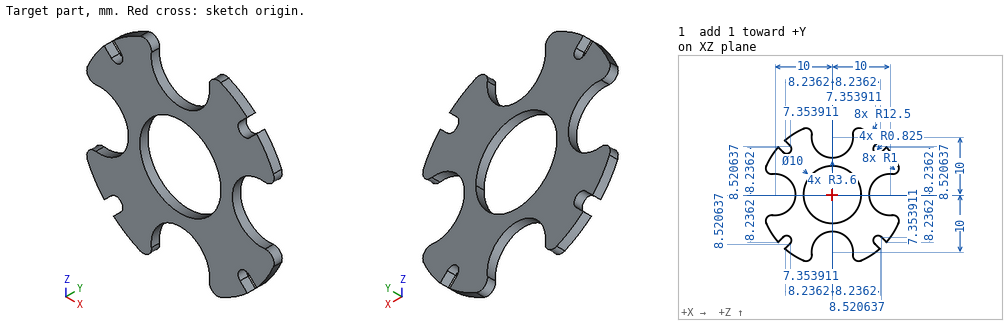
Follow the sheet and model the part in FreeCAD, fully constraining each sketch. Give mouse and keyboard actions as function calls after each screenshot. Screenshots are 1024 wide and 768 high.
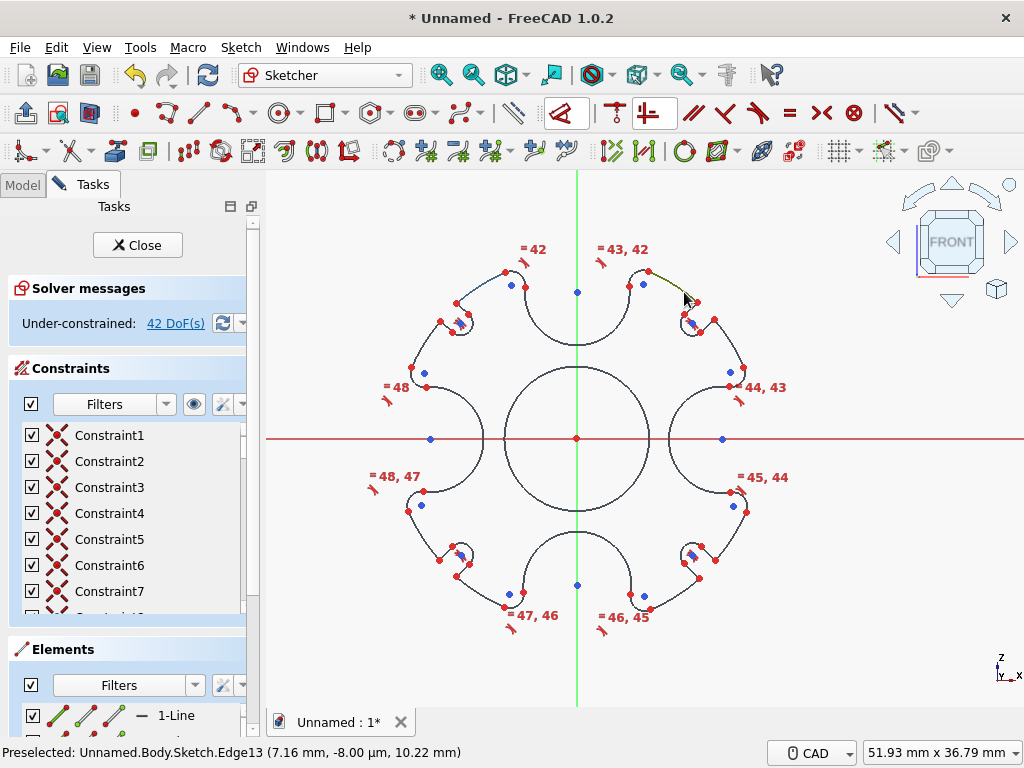
click(737, 352)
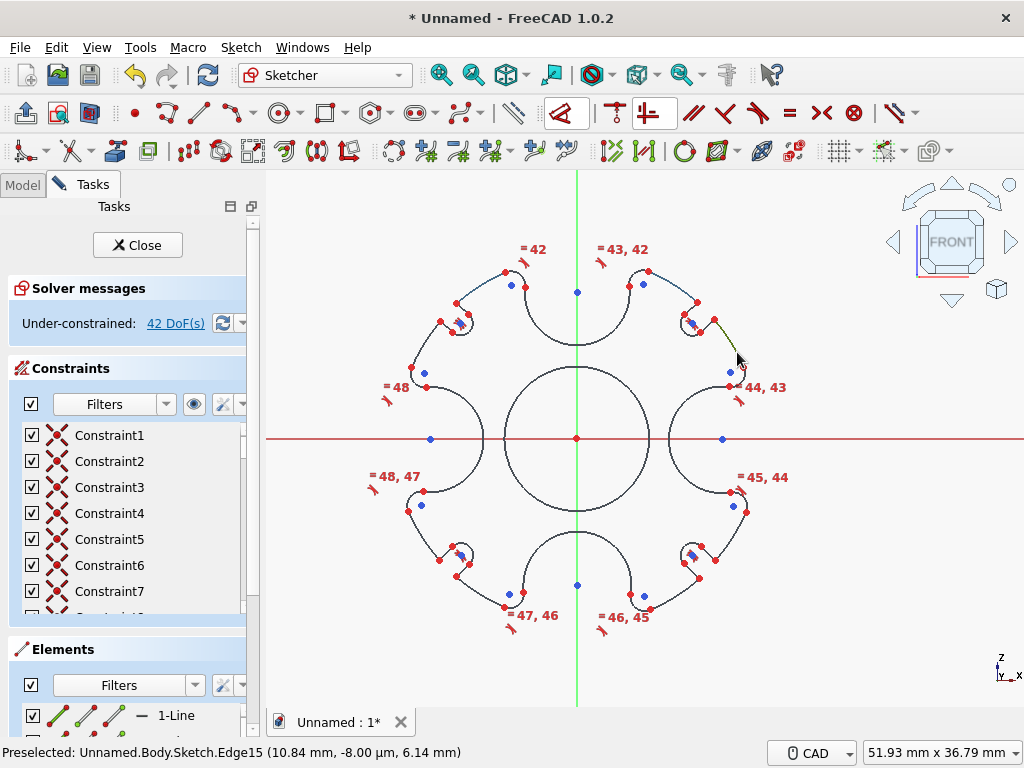
click(726, 547)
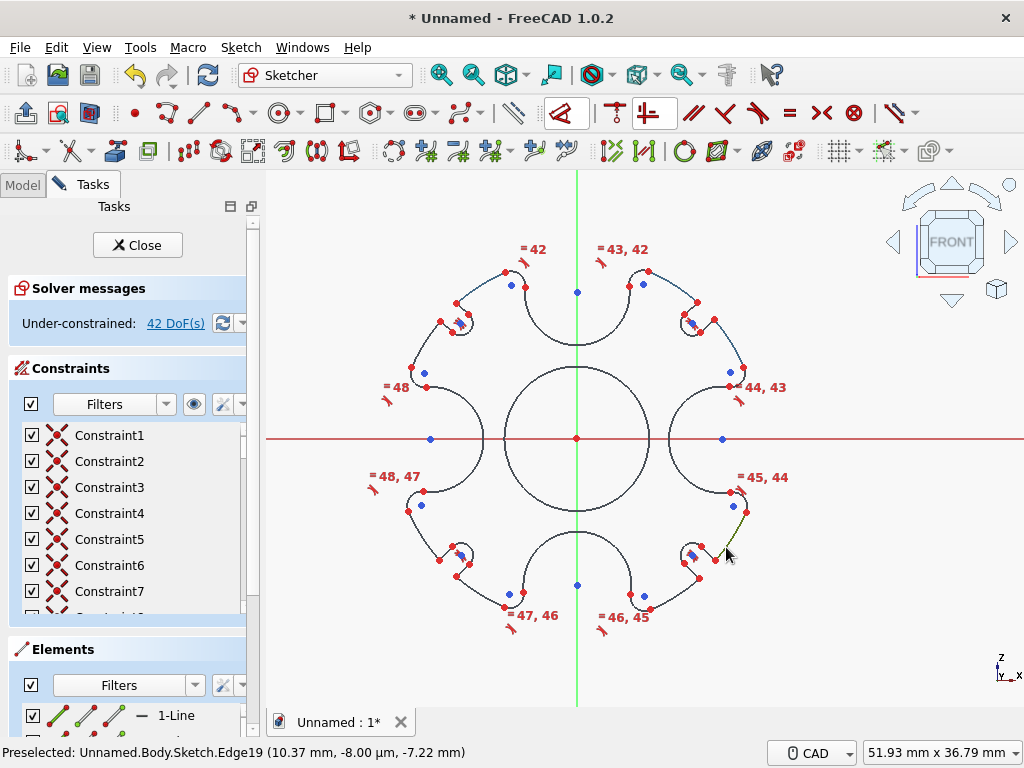
click(666, 602)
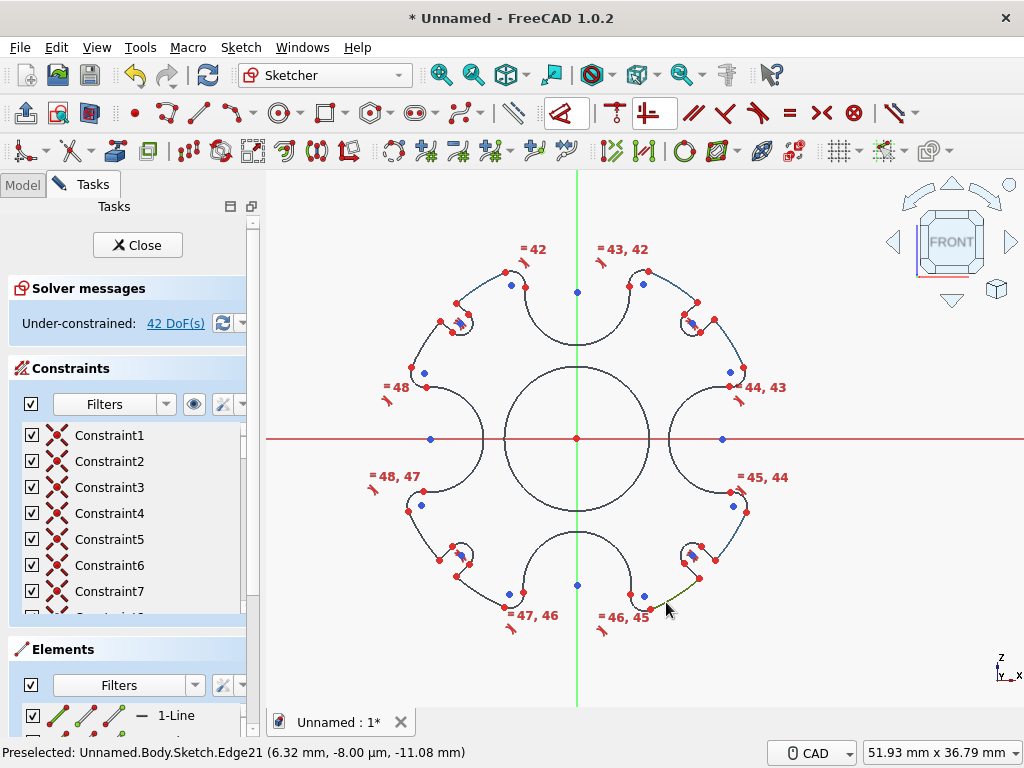
click(470, 588)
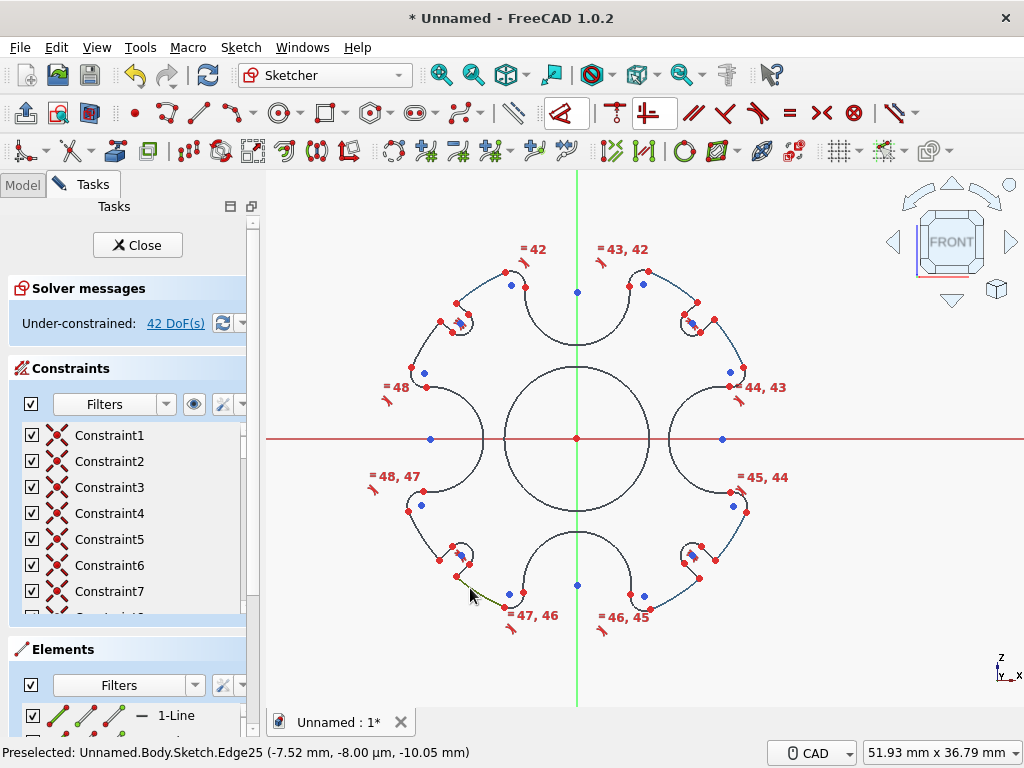
click(416, 527)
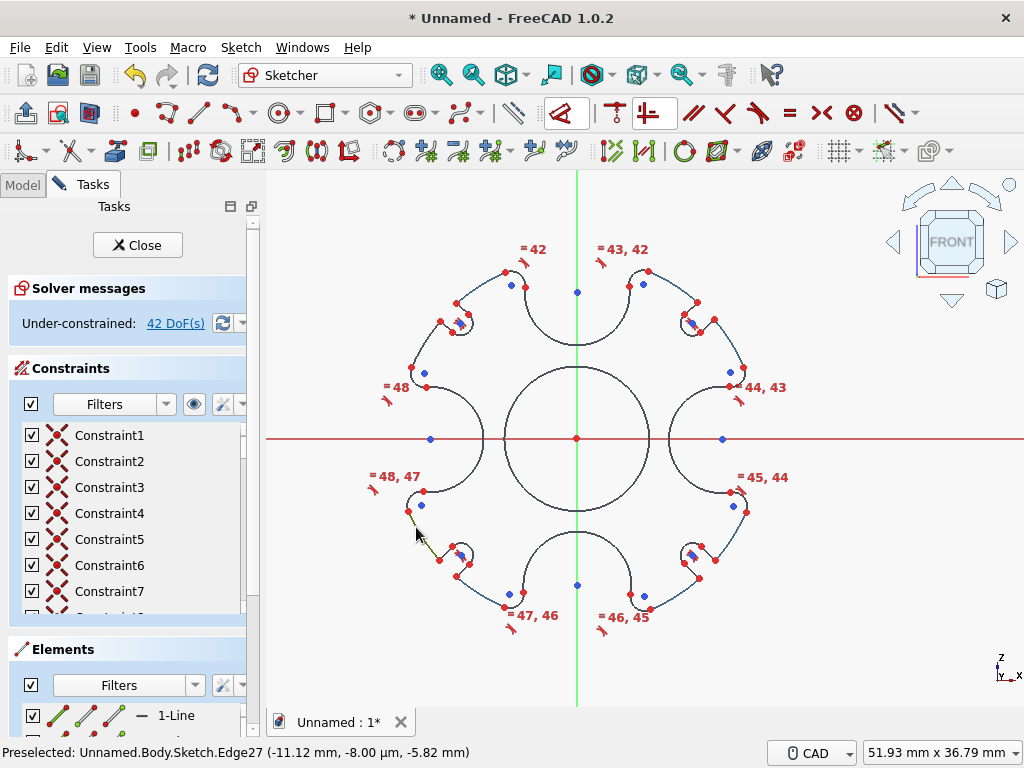
click(431, 334)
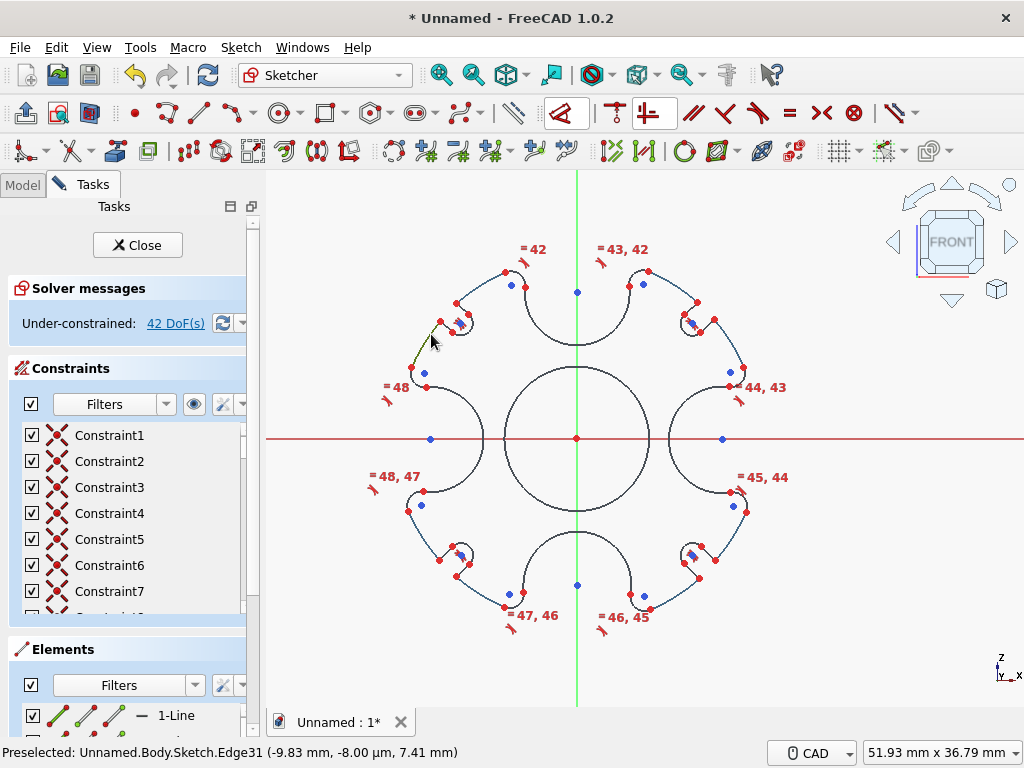
key(e)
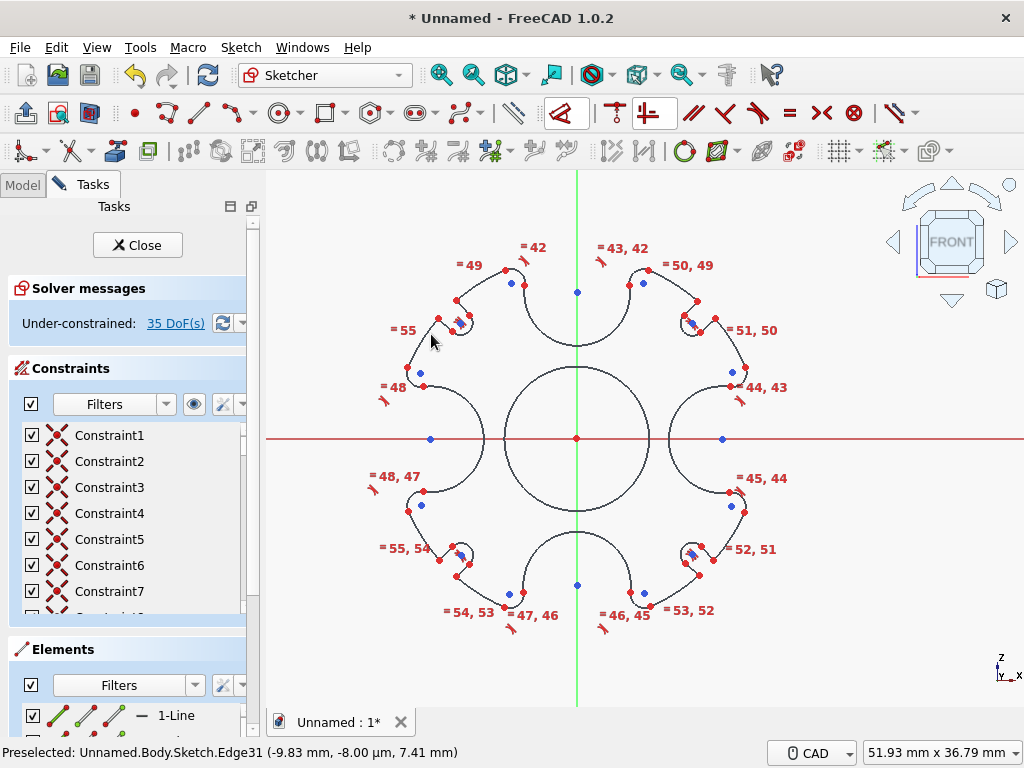
click(544, 334)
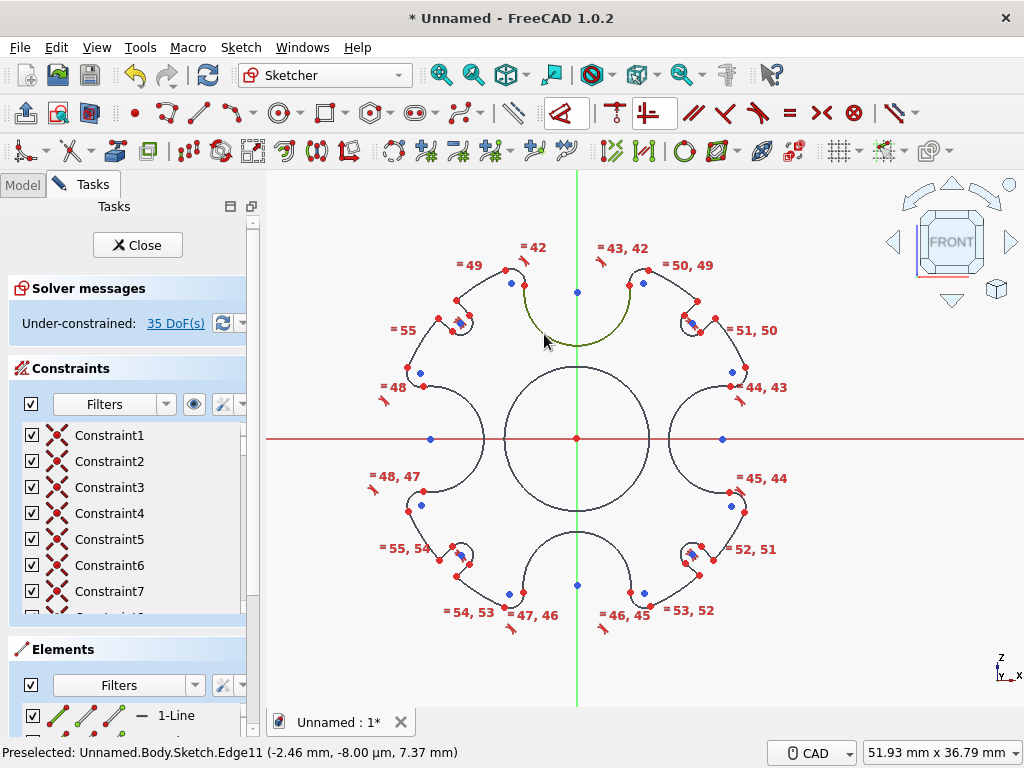
click(681, 406)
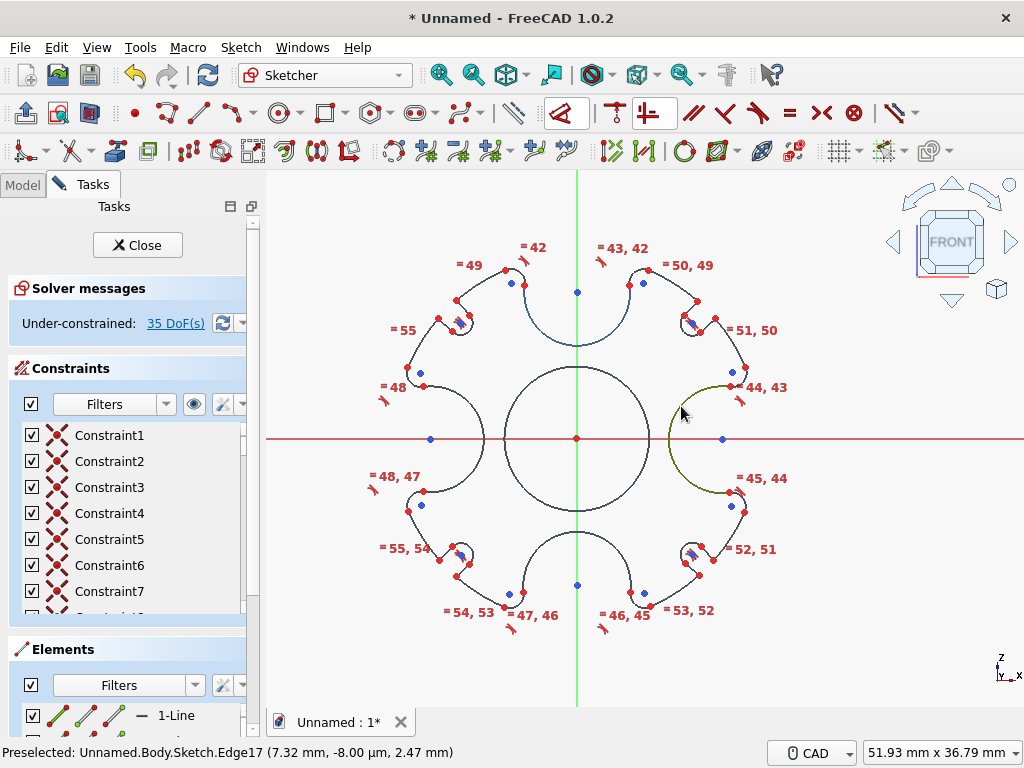
click(611, 544)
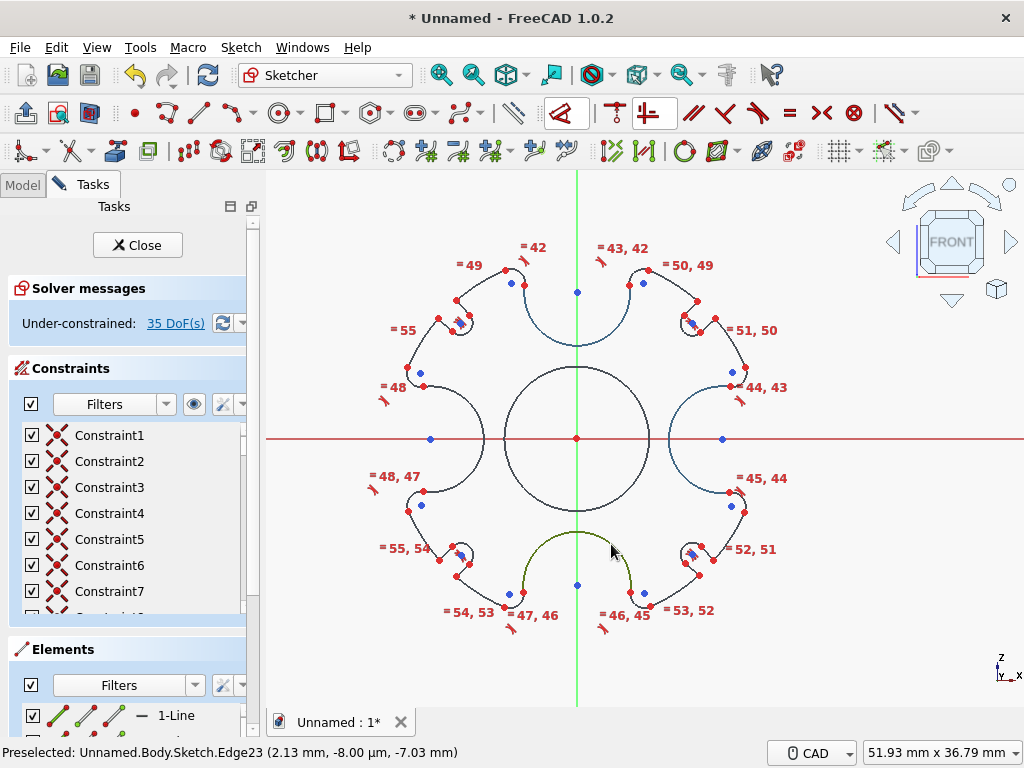
click(472, 473)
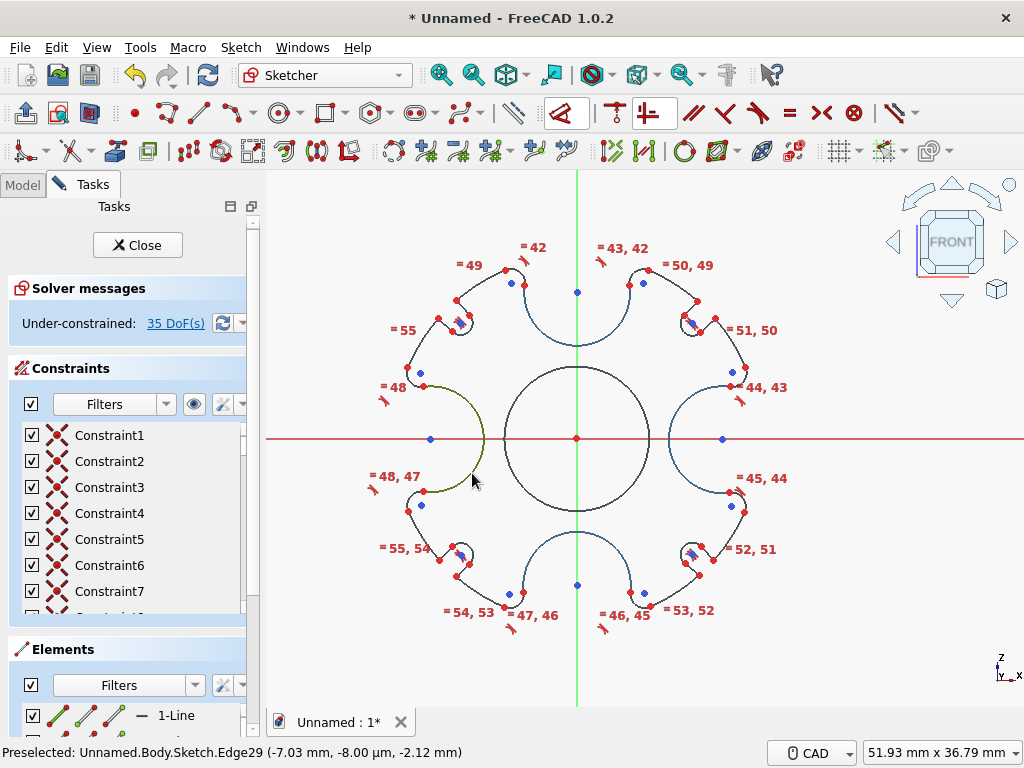
click(790, 114)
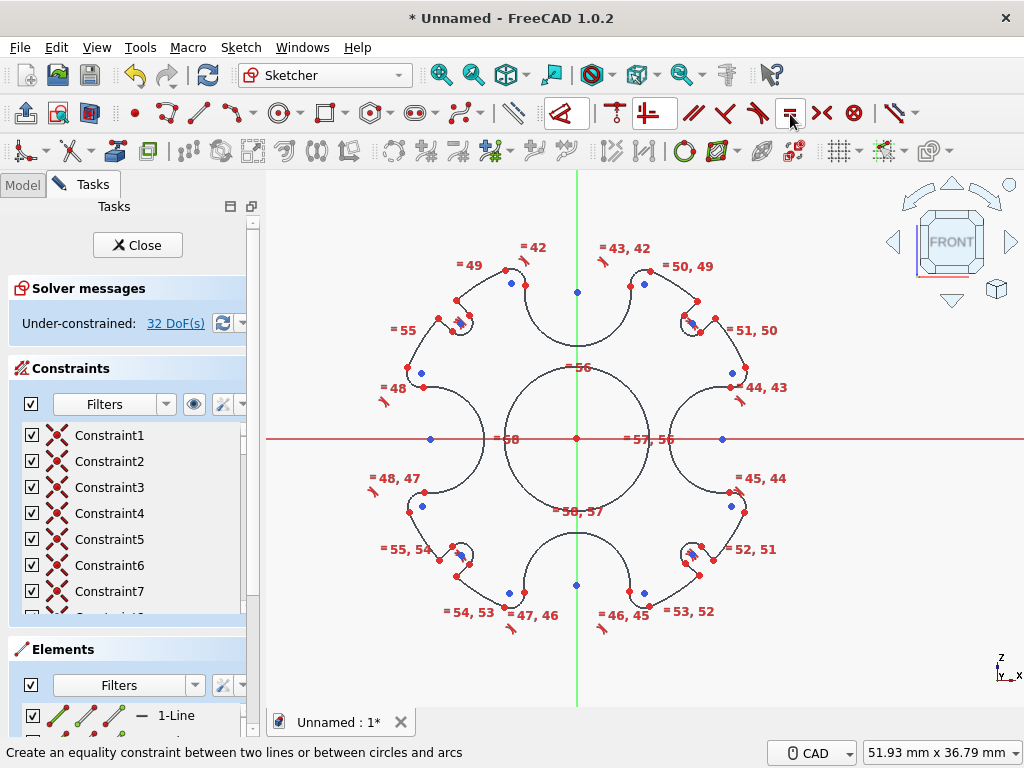
scroll(681, 326, up, 2)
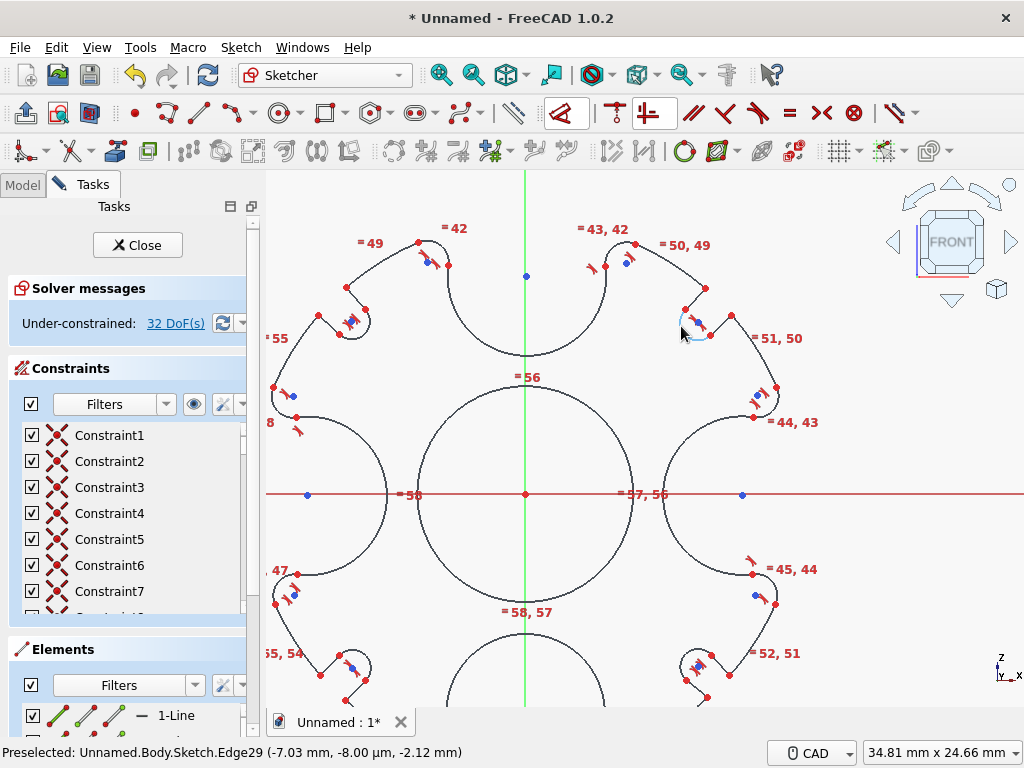
click(680, 325)